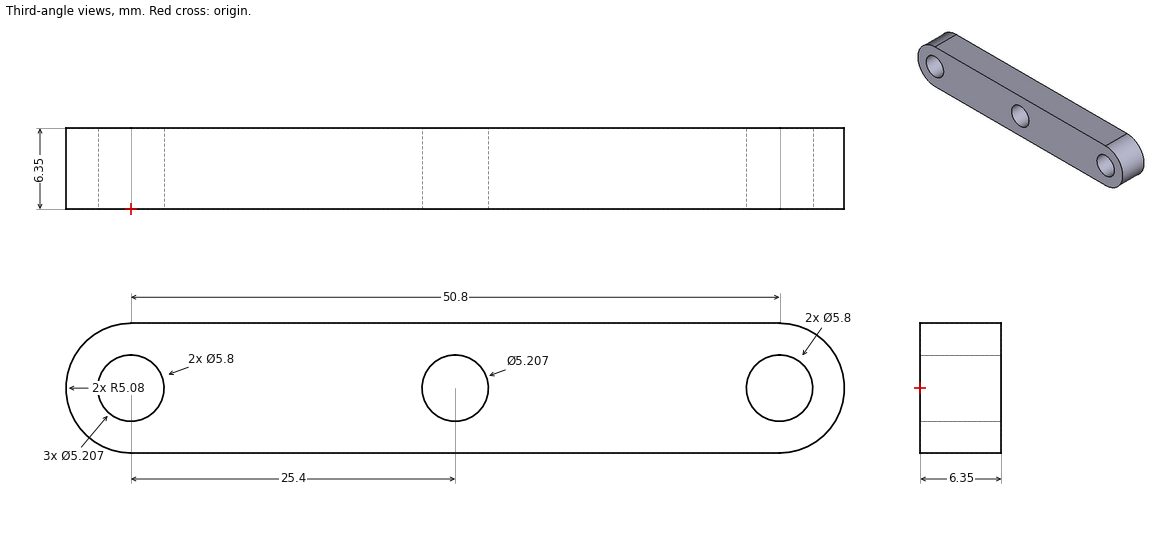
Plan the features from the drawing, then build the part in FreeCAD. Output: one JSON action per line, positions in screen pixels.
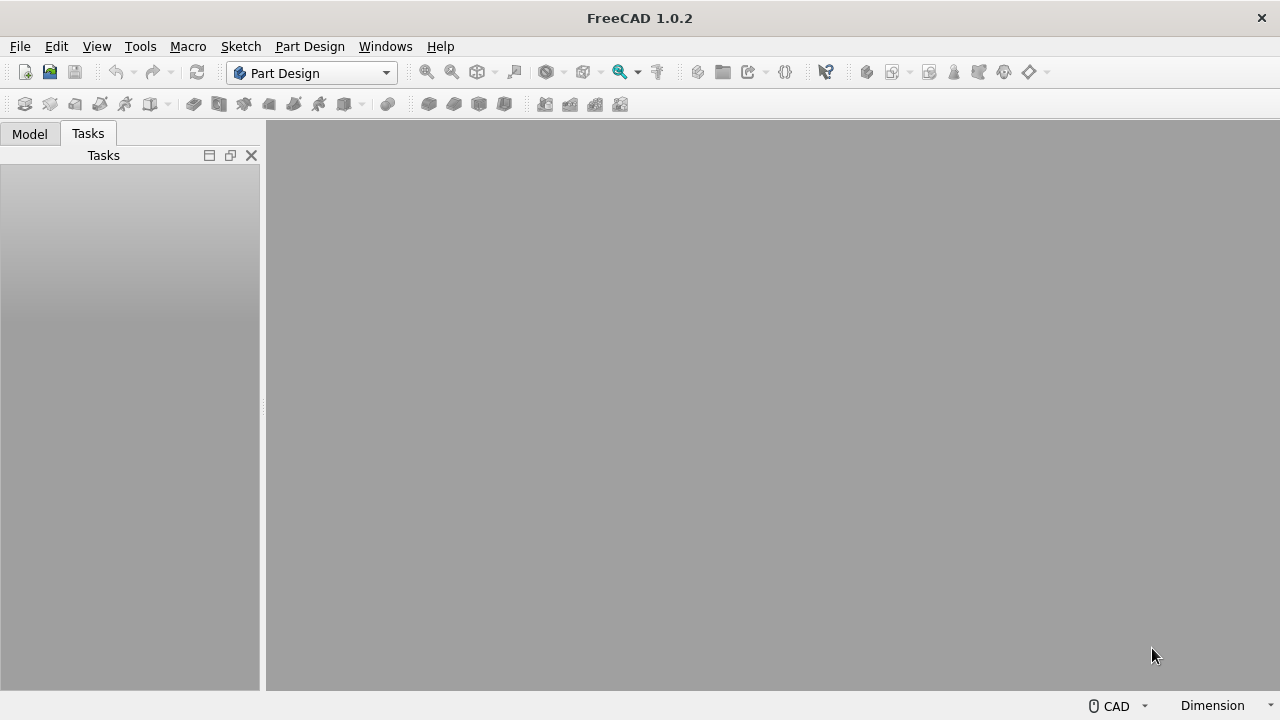
{"action": "left_click", "coordinate": [25, 72]}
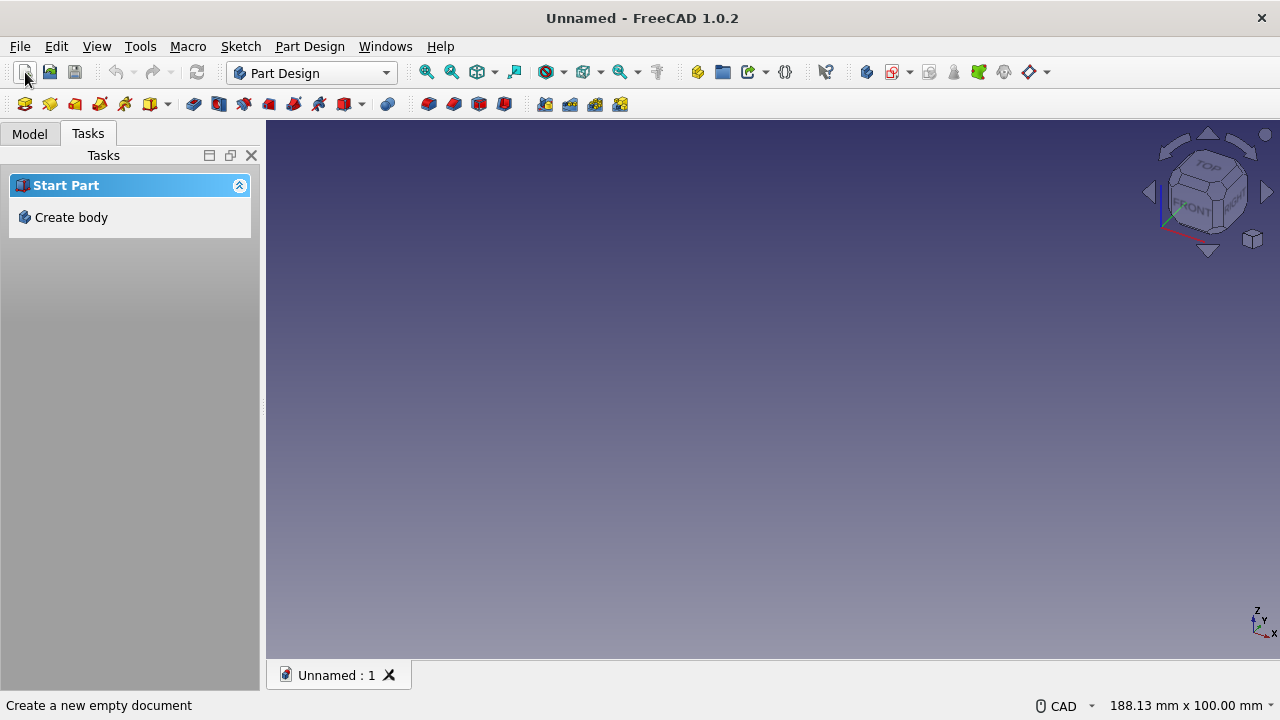
{"action": "left_click", "coordinate": [892, 72]}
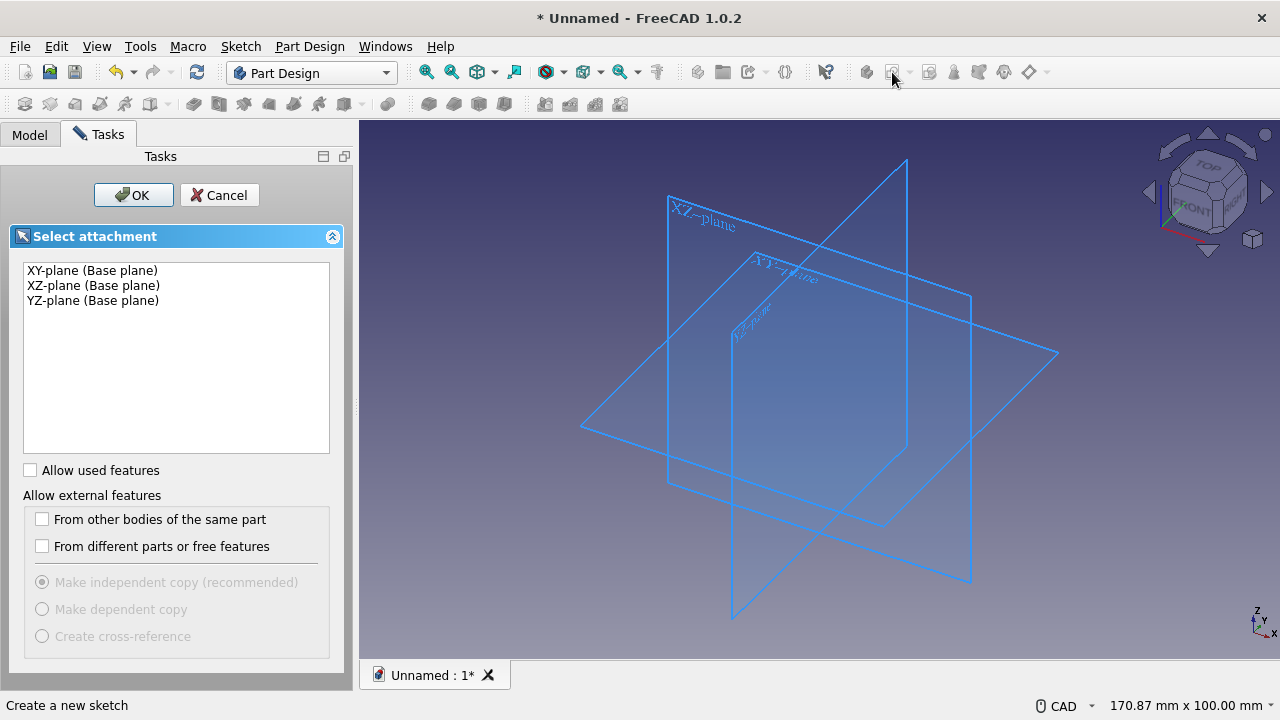
{"action": "left_click", "coordinate": [84, 286]}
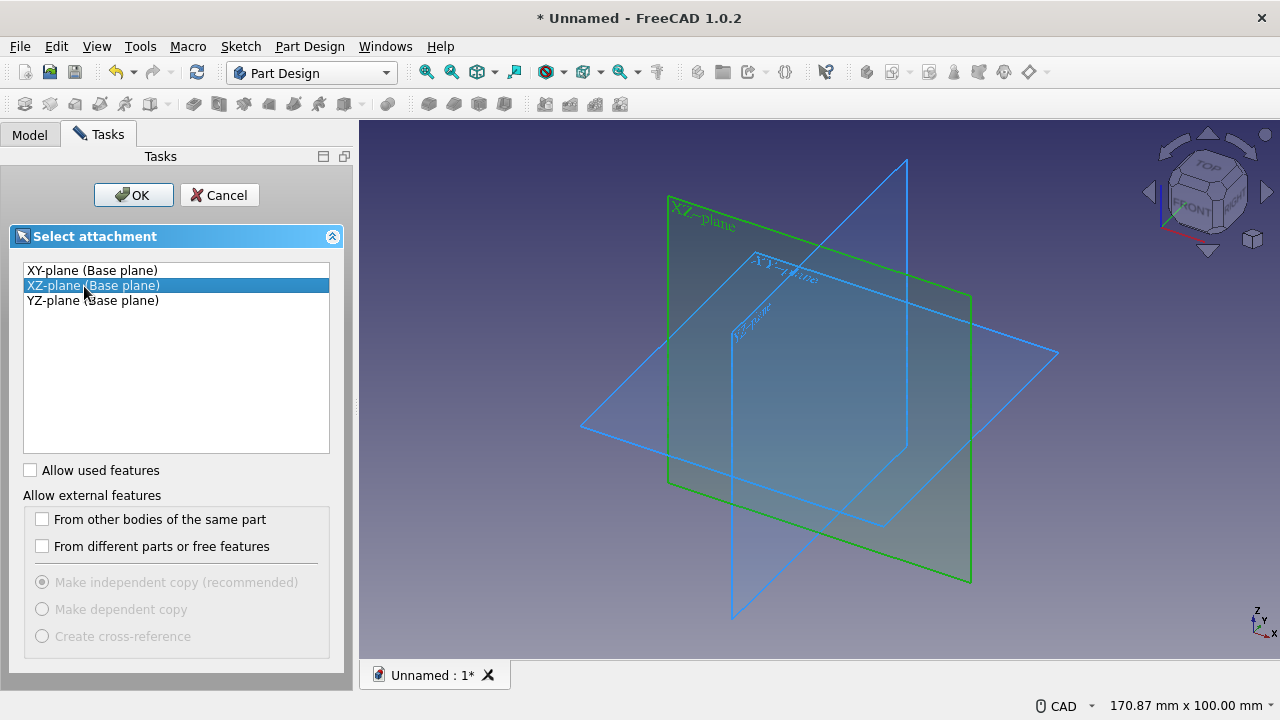
{"action": "left_click", "coordinate": [134, 195]}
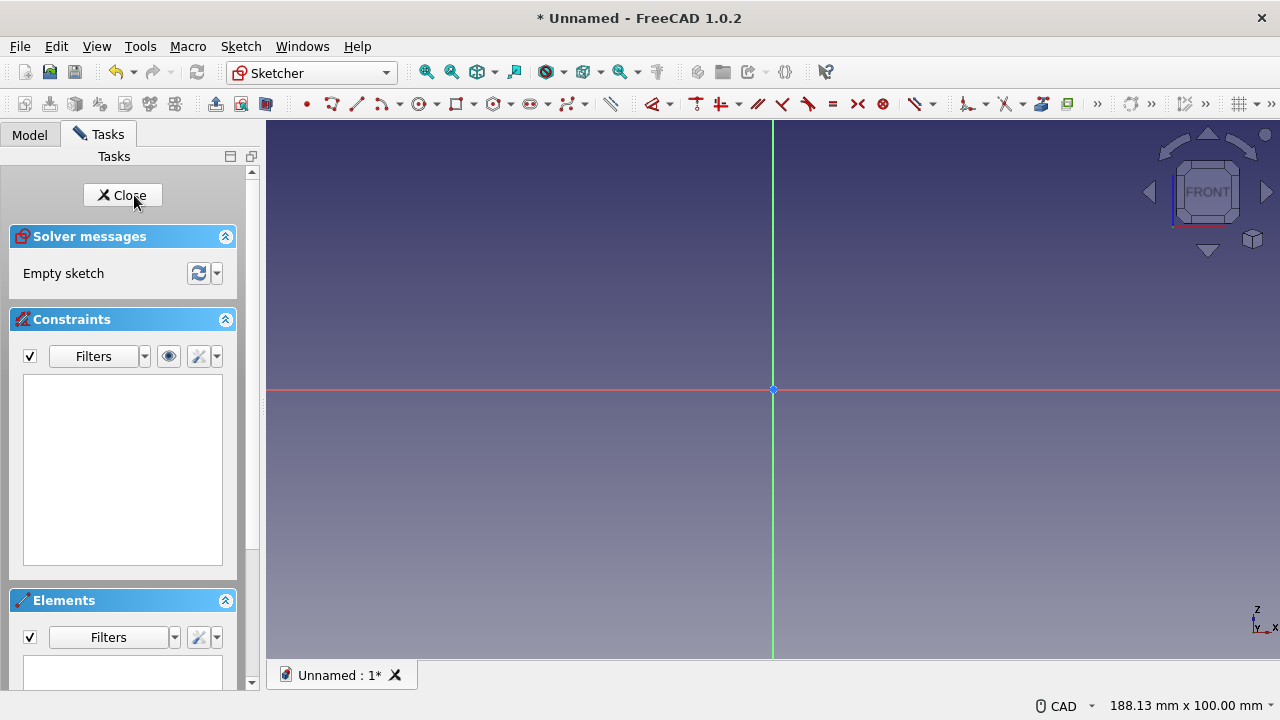
{"action": "scroll", "coordinate": [1115, 389], "scroll_direction": "up", "scroll_amount": 3}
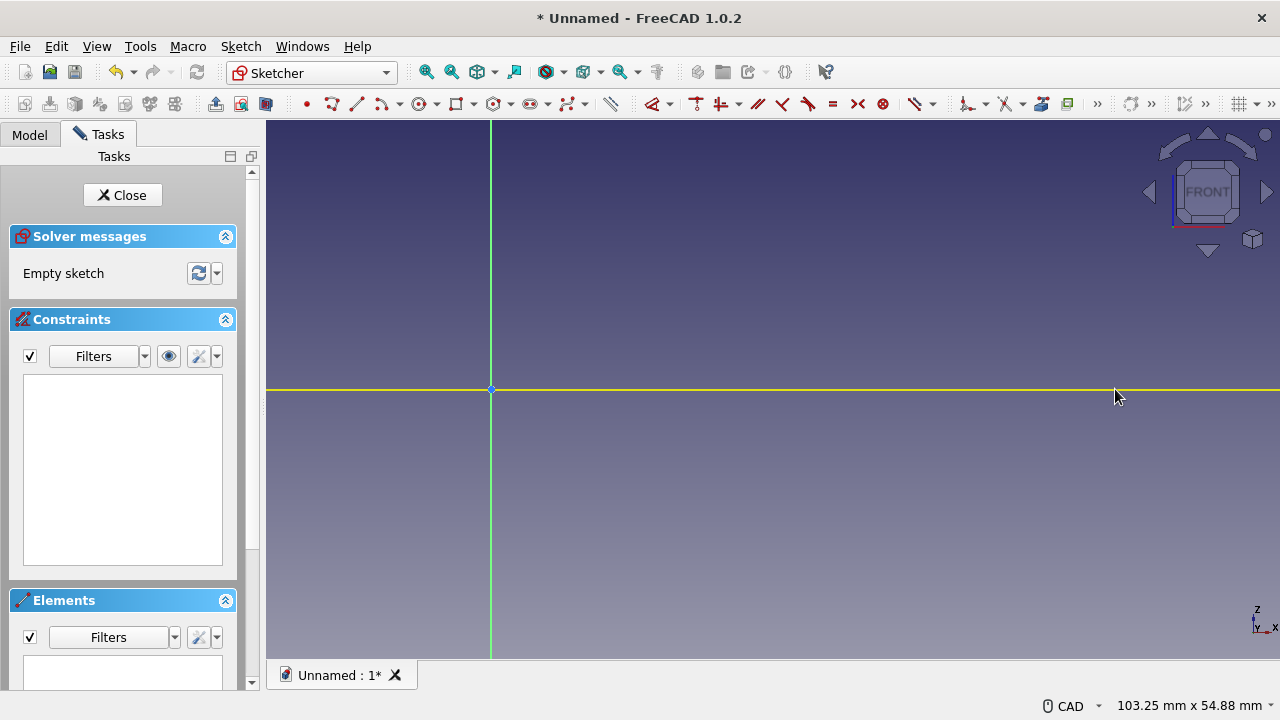
{"action": "key", "text": "g s"}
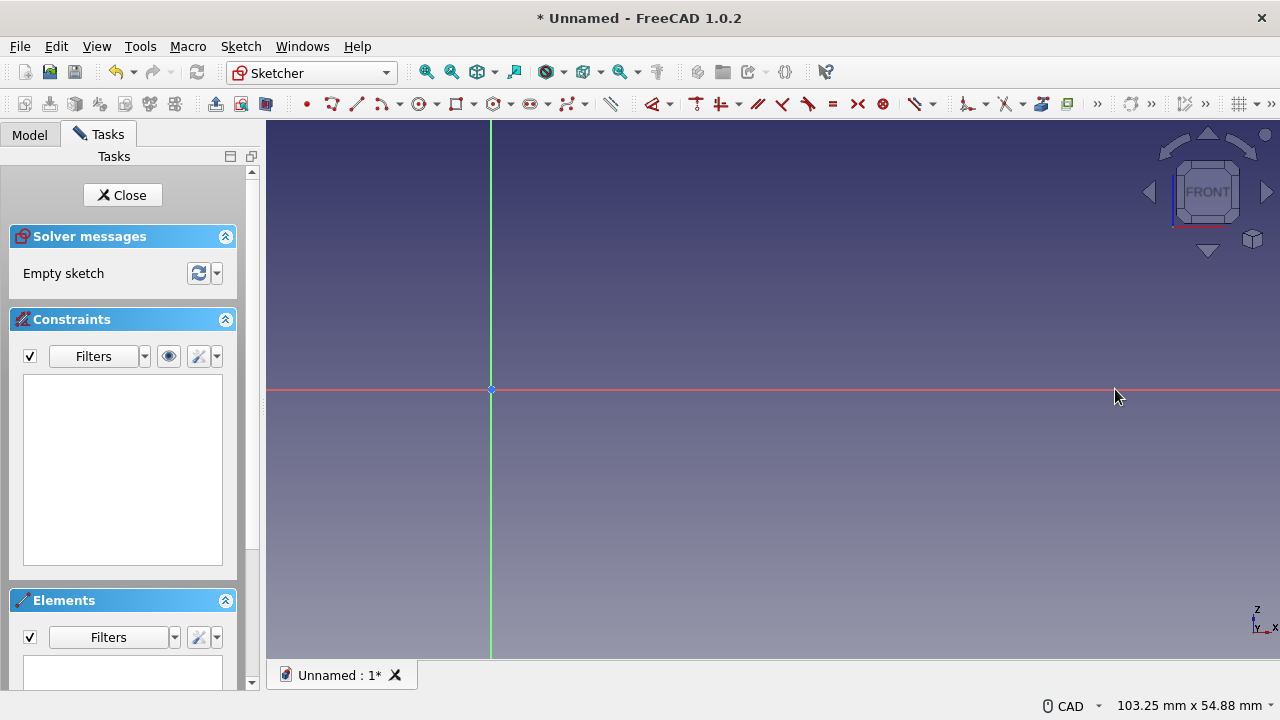
{"action": "left_click", "coordinate": [491, 390]}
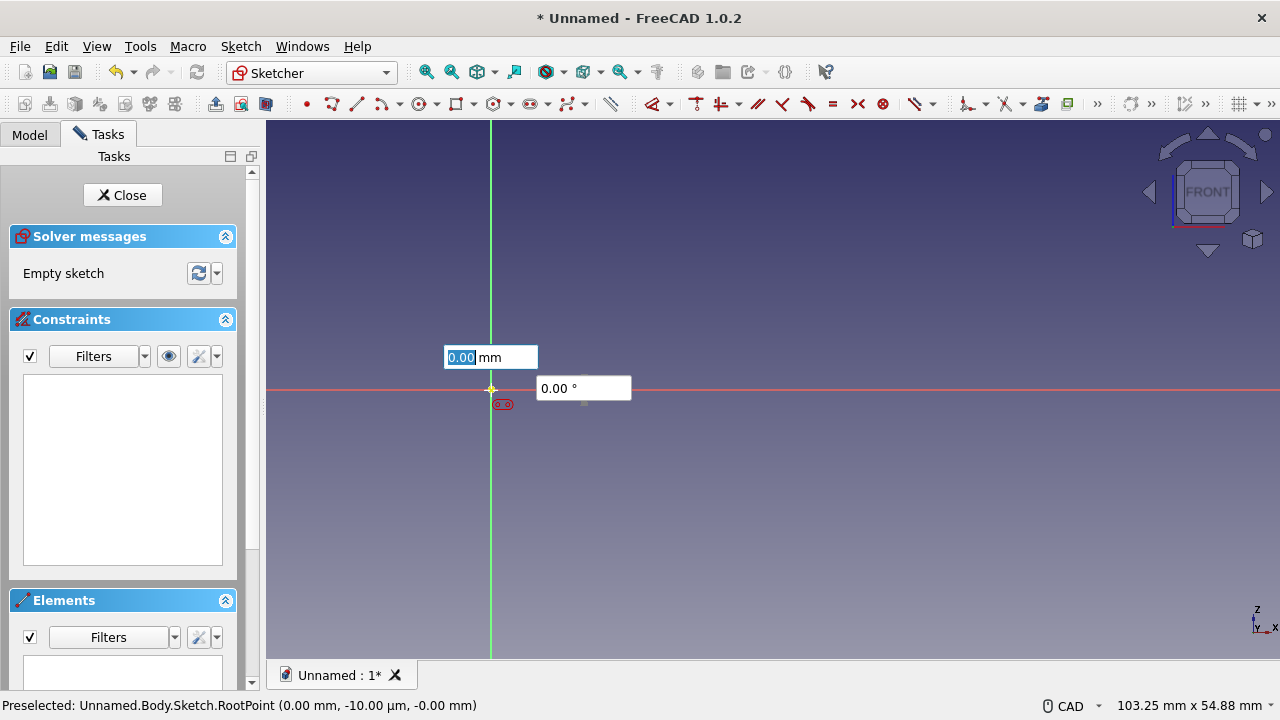
{"action": "left_click", "coordinate": [990, 380]}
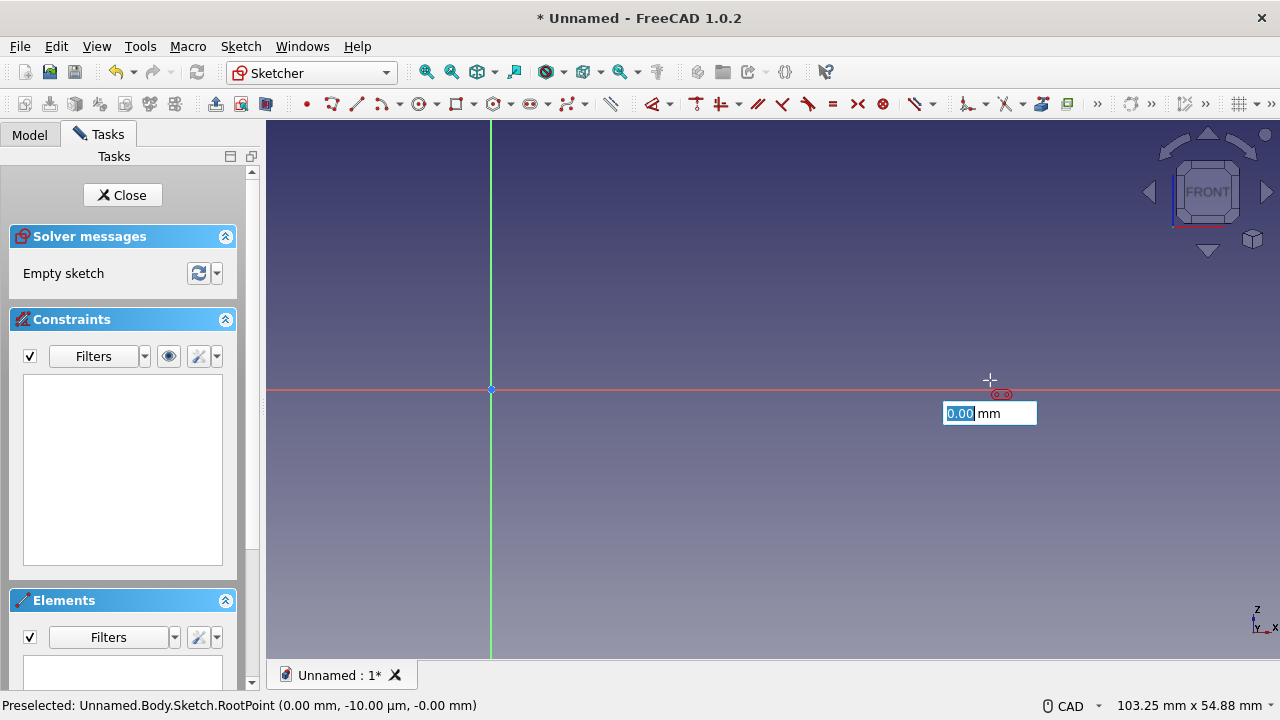
{"action": "left_click", "coordinate": [741, 439]}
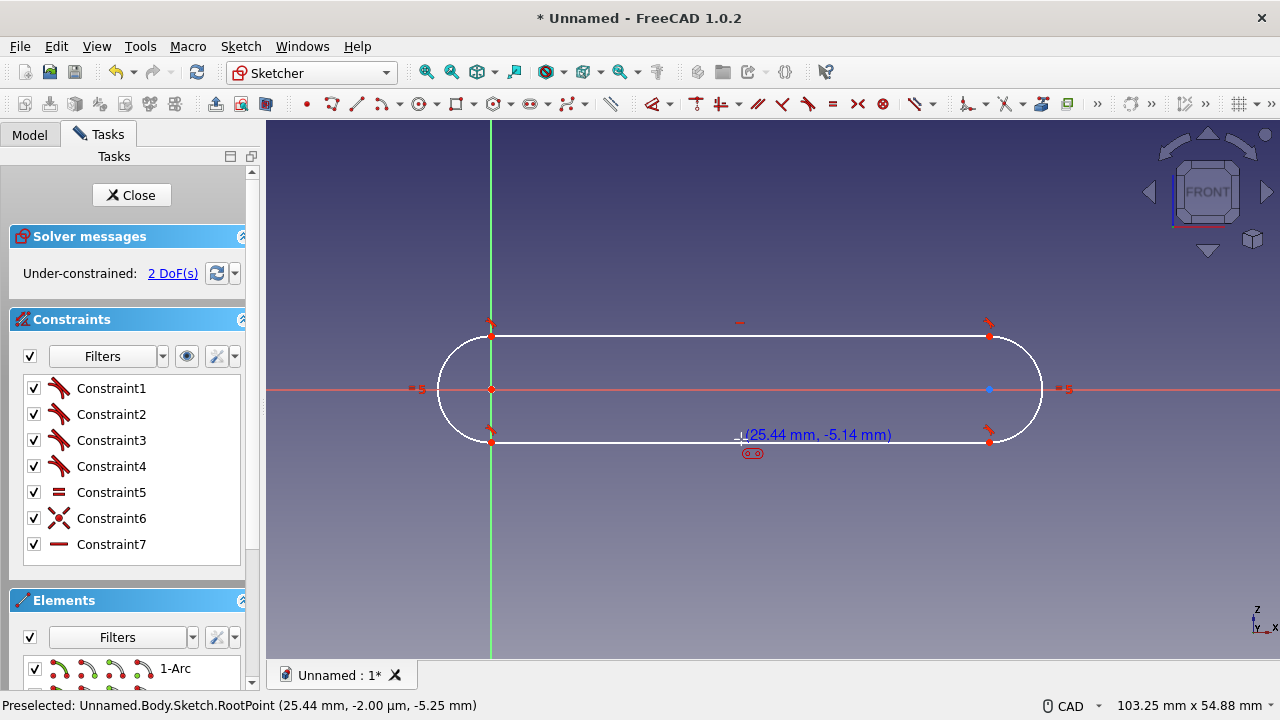
{"action": "left_click", "coordinate": [418, 104]}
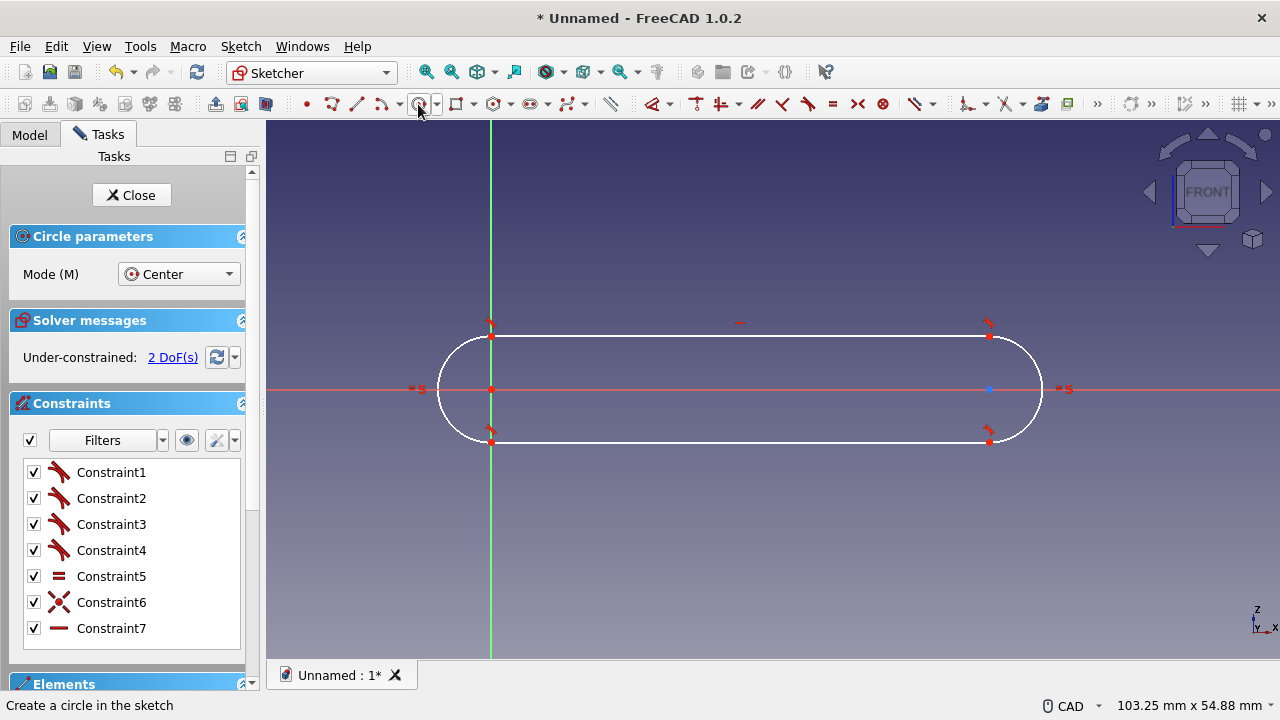
{"action": "left_click", "coordinate": [990, 380]}
{"action": "mouse_move", "coordinate": [1010, 369]}